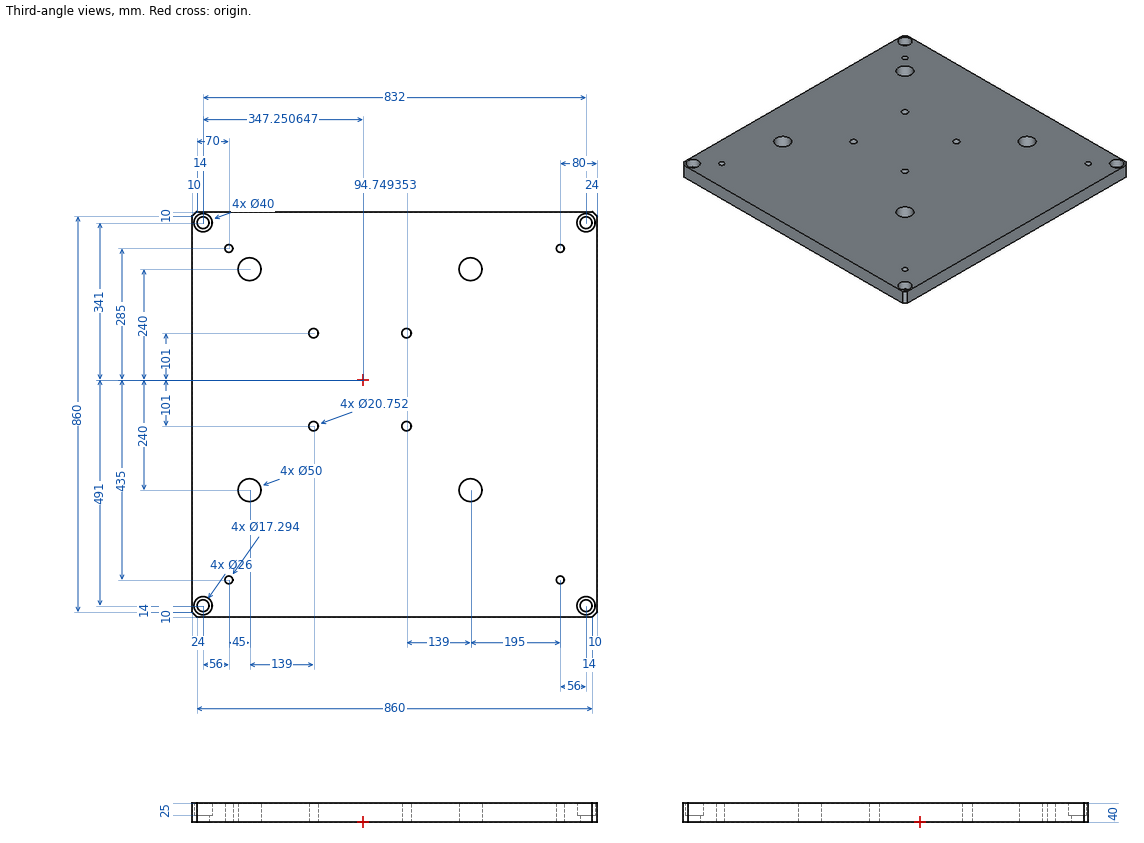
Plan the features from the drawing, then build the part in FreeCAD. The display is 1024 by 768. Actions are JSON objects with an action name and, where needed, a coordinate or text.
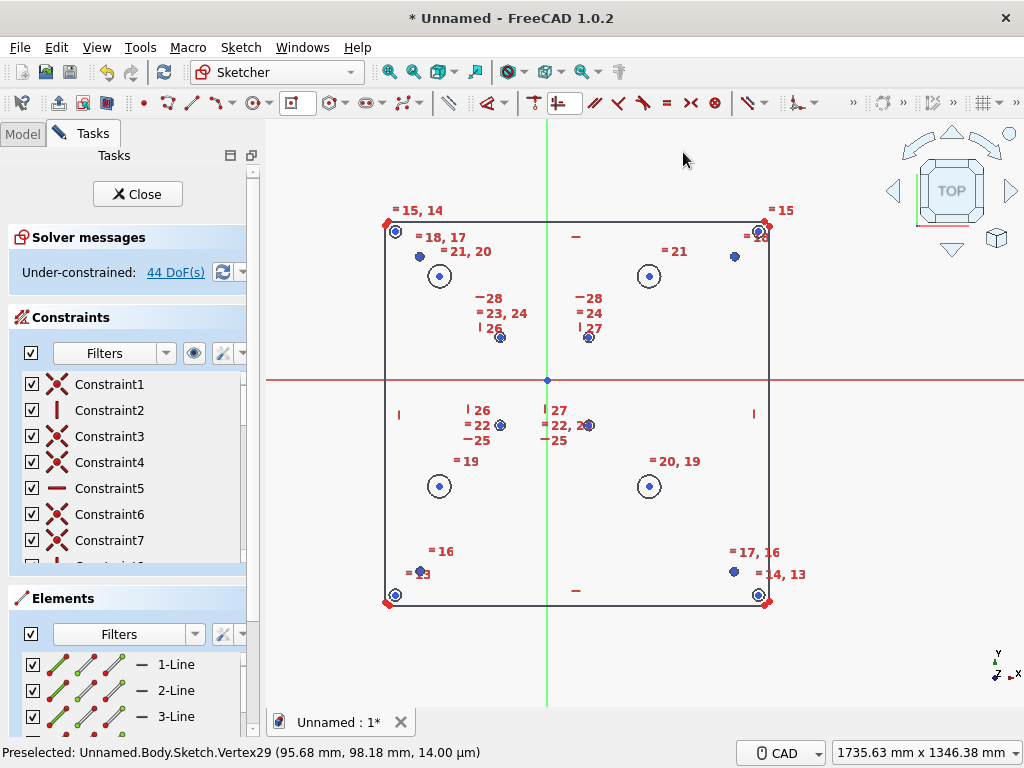
{"action": "scroll", "coordinate": [400, 599], "scroll_direction": "up", "scroll_amount": 7}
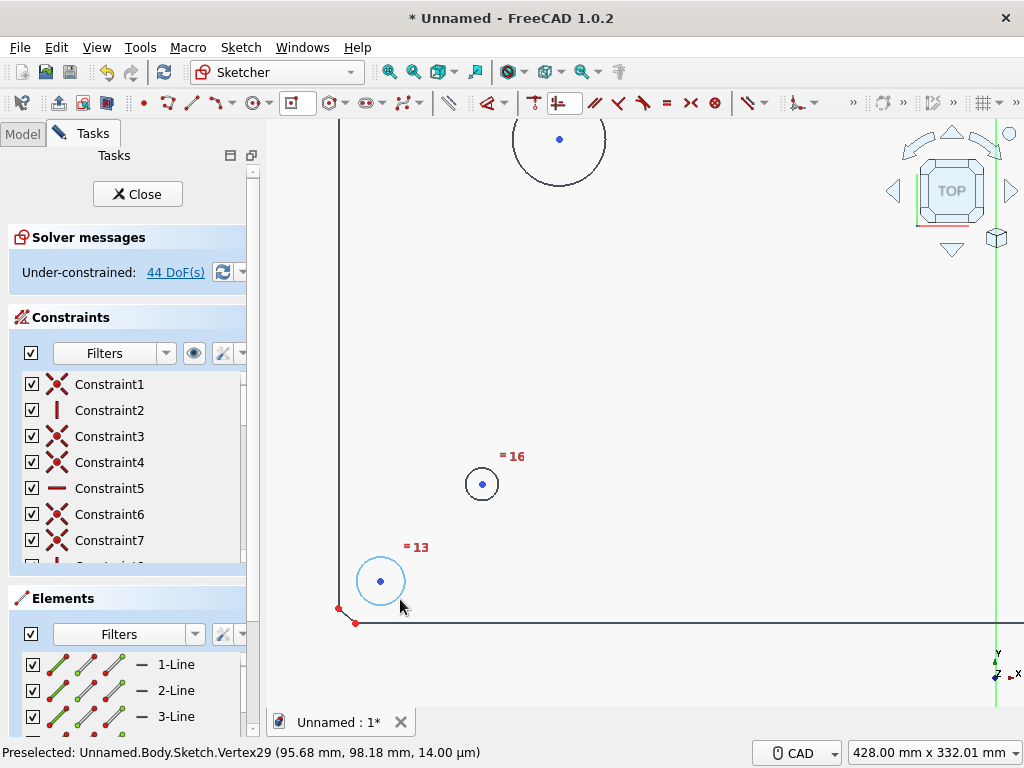
{"action": "left_click", "coordinate": [398, 598]}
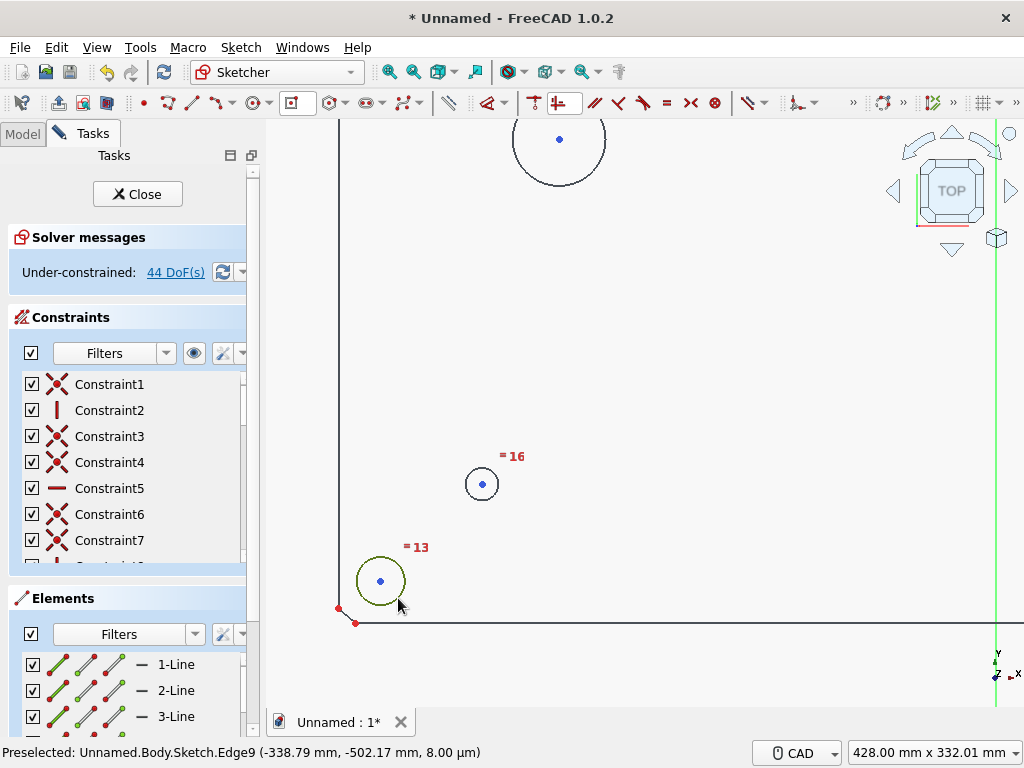
{"action": "left_click", "coordinate": [506, 104]}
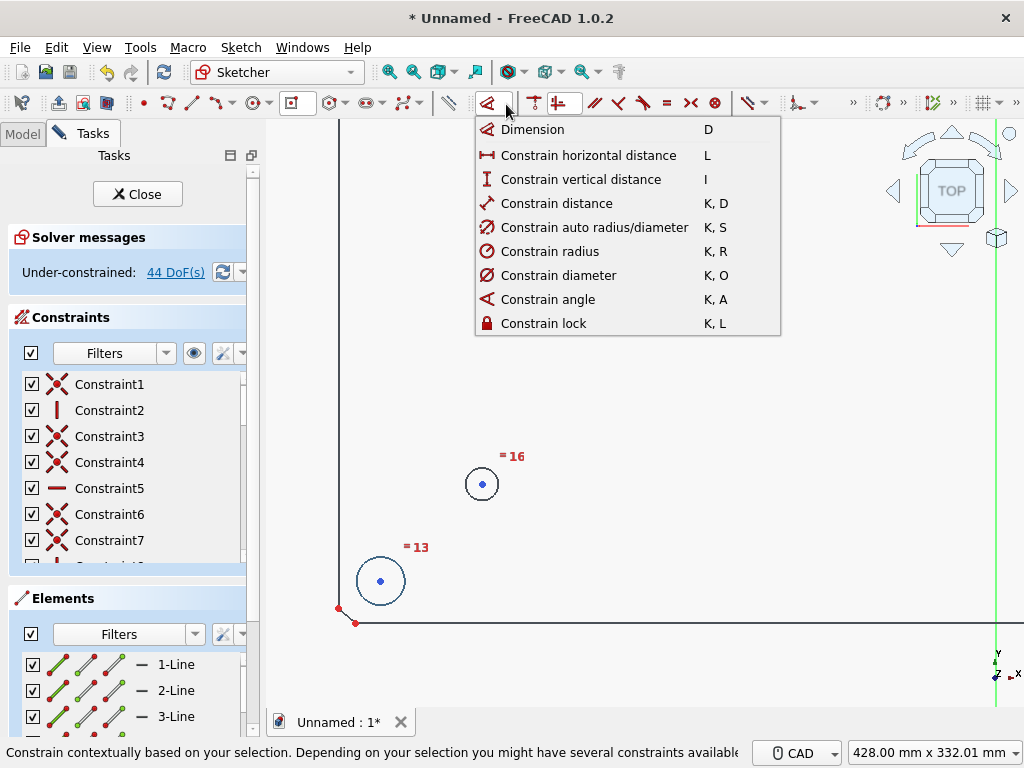
{"action": "left_click", "coordinate": [628, 275]}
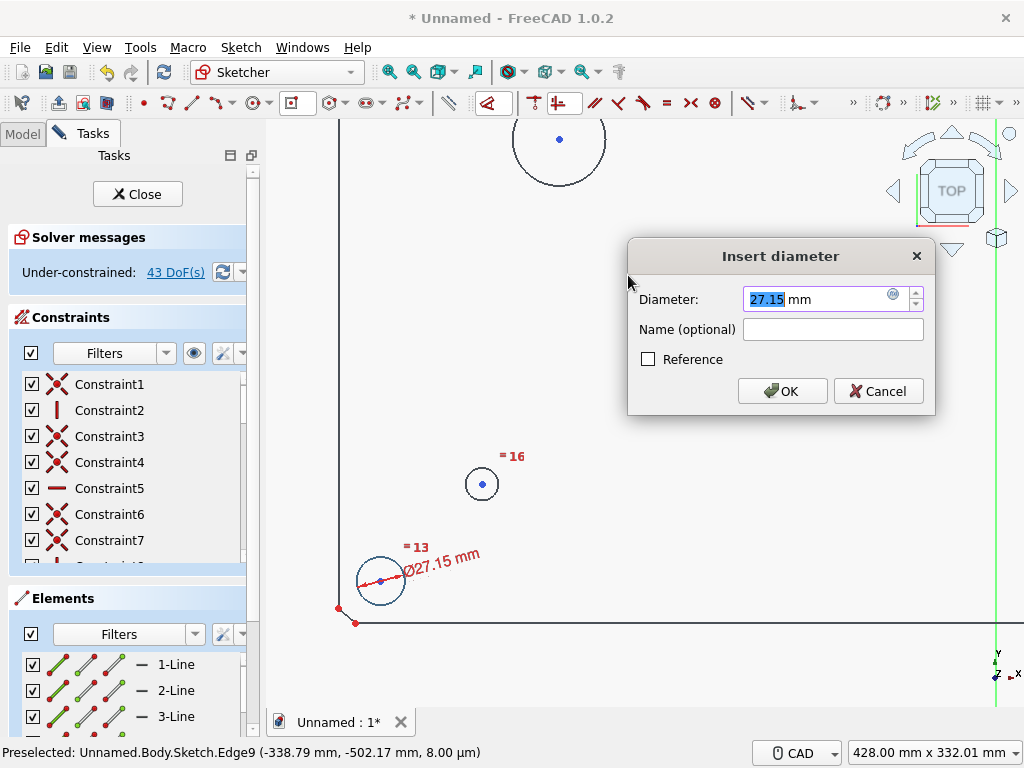
{"action": "type", "text": "26"}
{"action": "key", "text": "Return"}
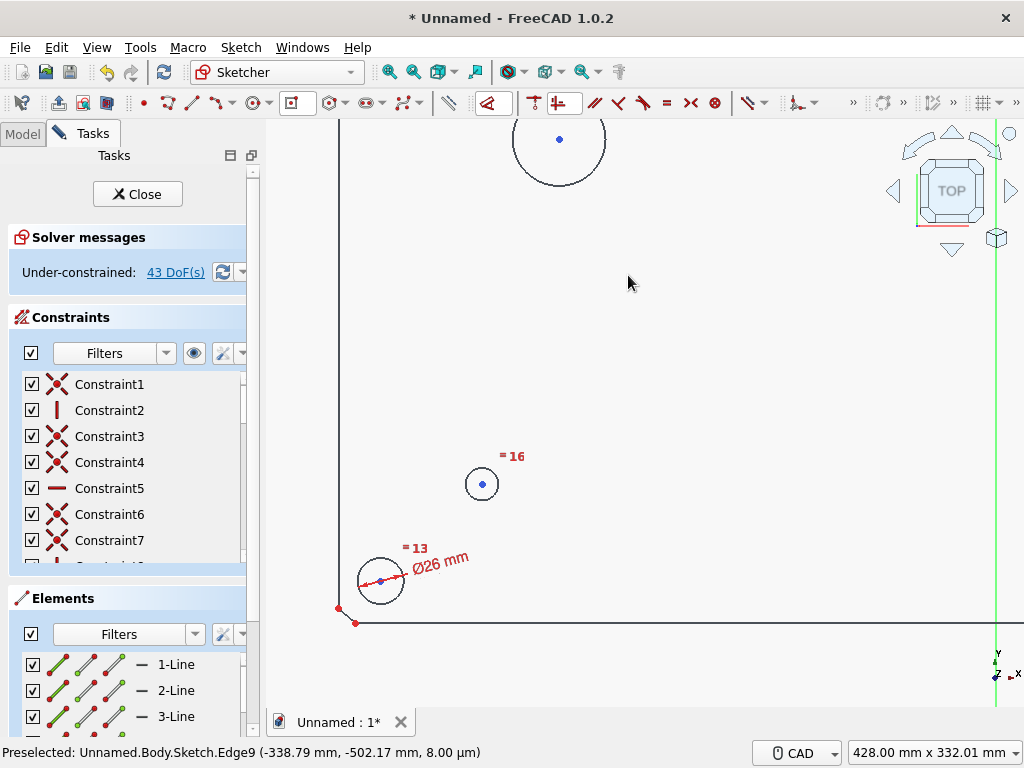
{"action": "scroll", "coordinate": [494, 473], "scroll_direction": "up", "scroll_amount": 2}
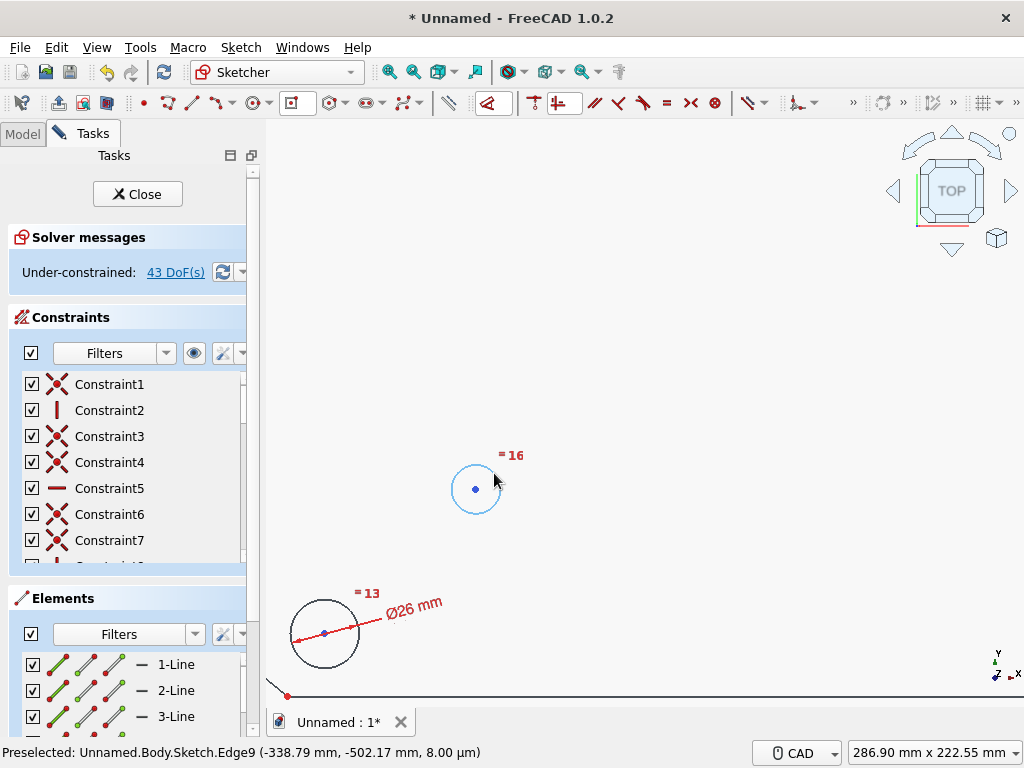
{"action": "left_click", "coordinate": [493, 472]}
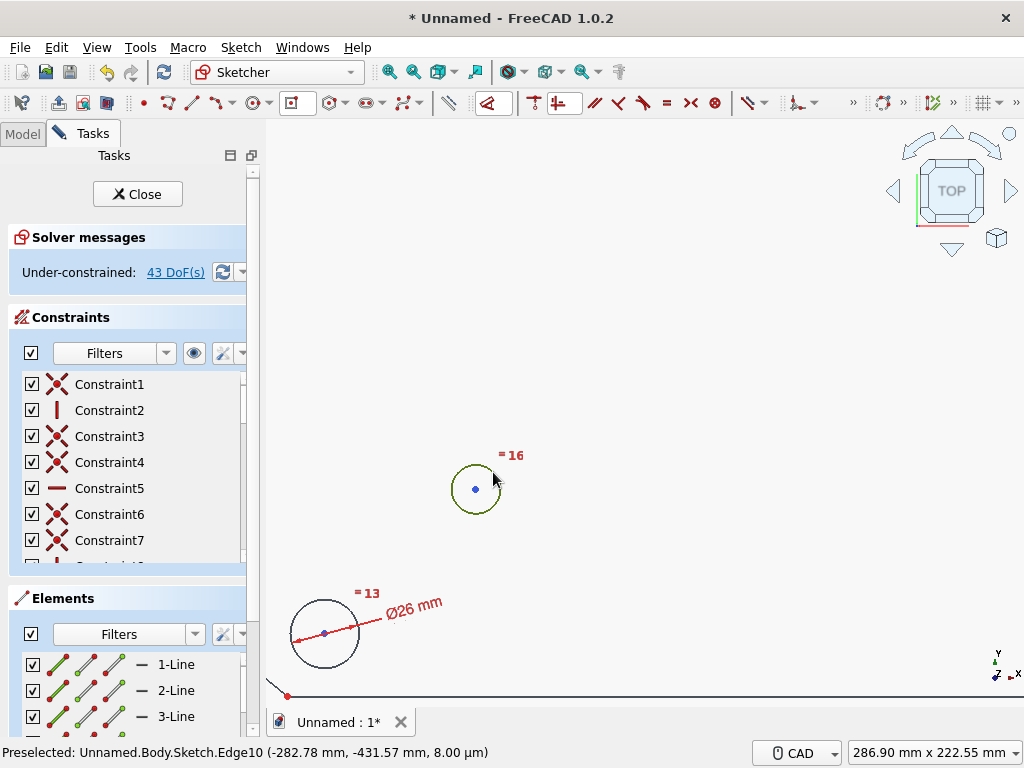
{"action": "key", "text": "k o"}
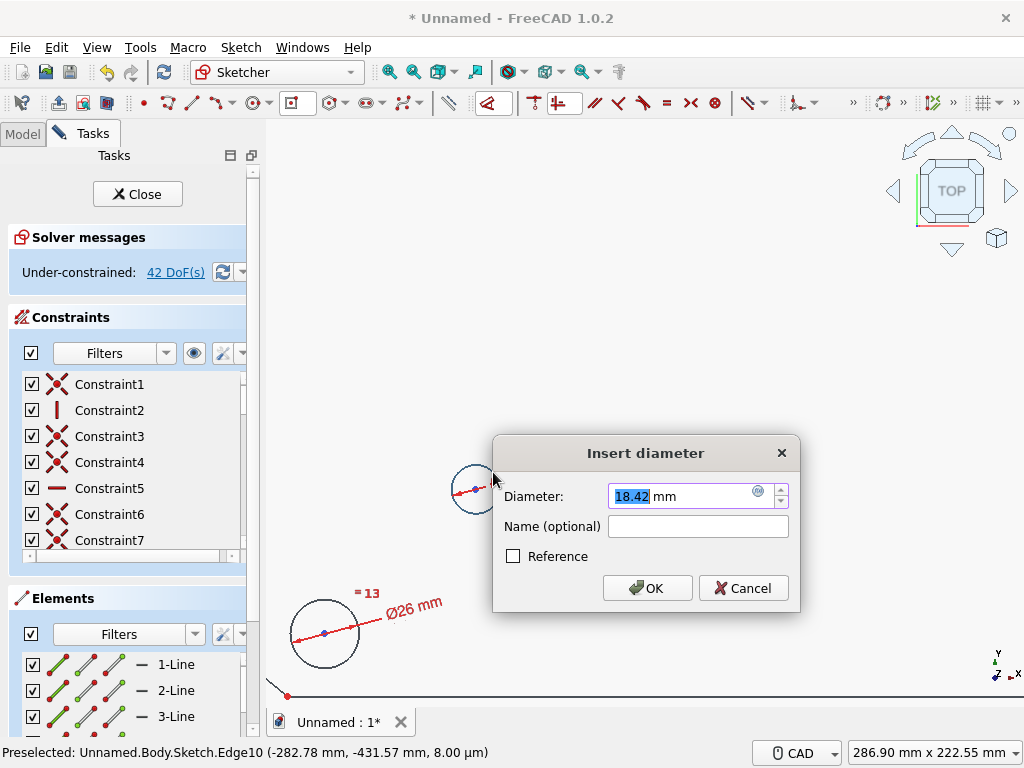
{"action": "type", "text": "17.294"}
{"action": "key", "text": "Return"}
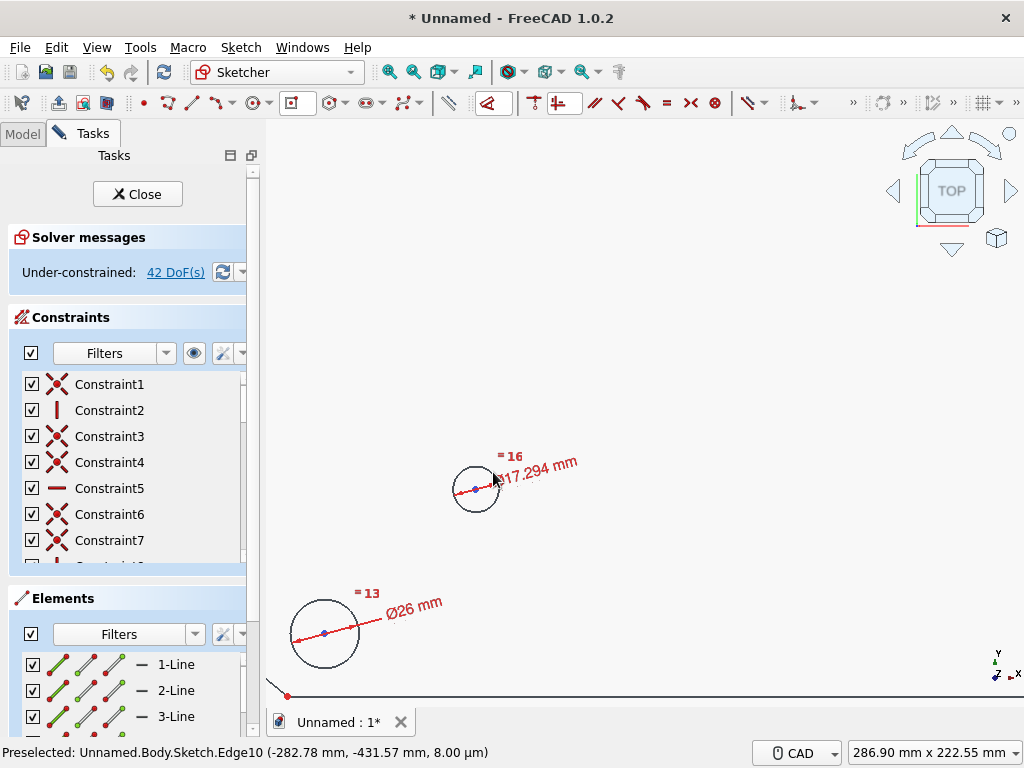
{"action": "scroll", "coordinate": [409, 587], "scroll_direction": "down", "scroll_amount": 9}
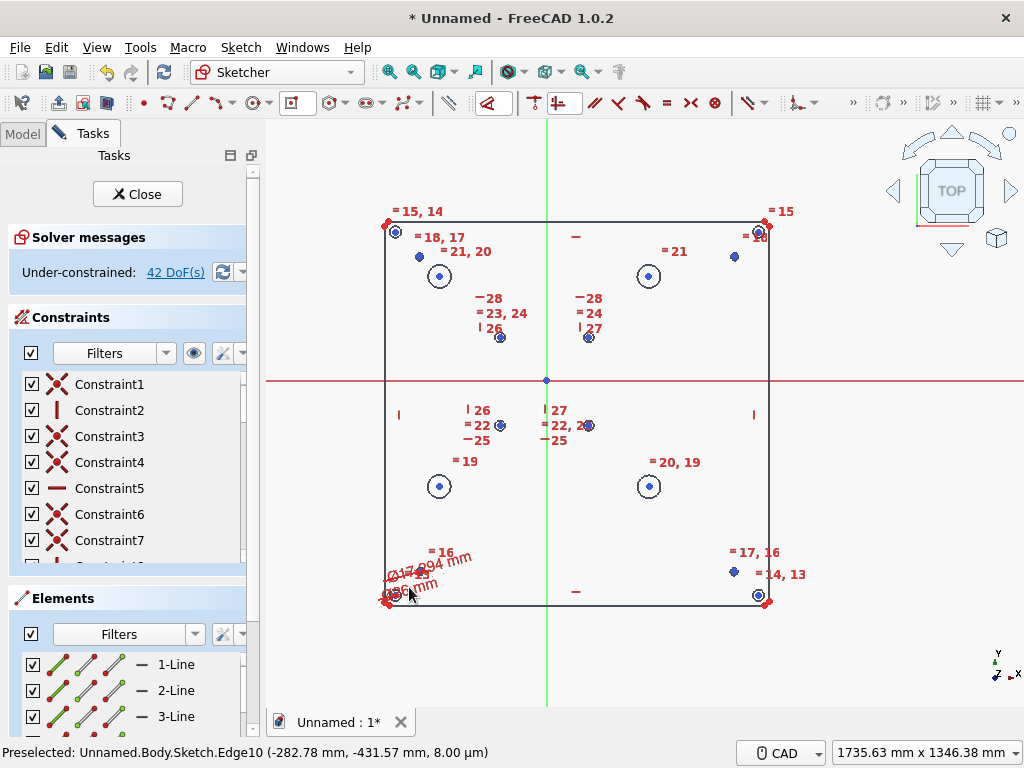
{"action": "scroll", "coordinate": [447, 478], "scroll_direction": "up", "scroll_amount": 3}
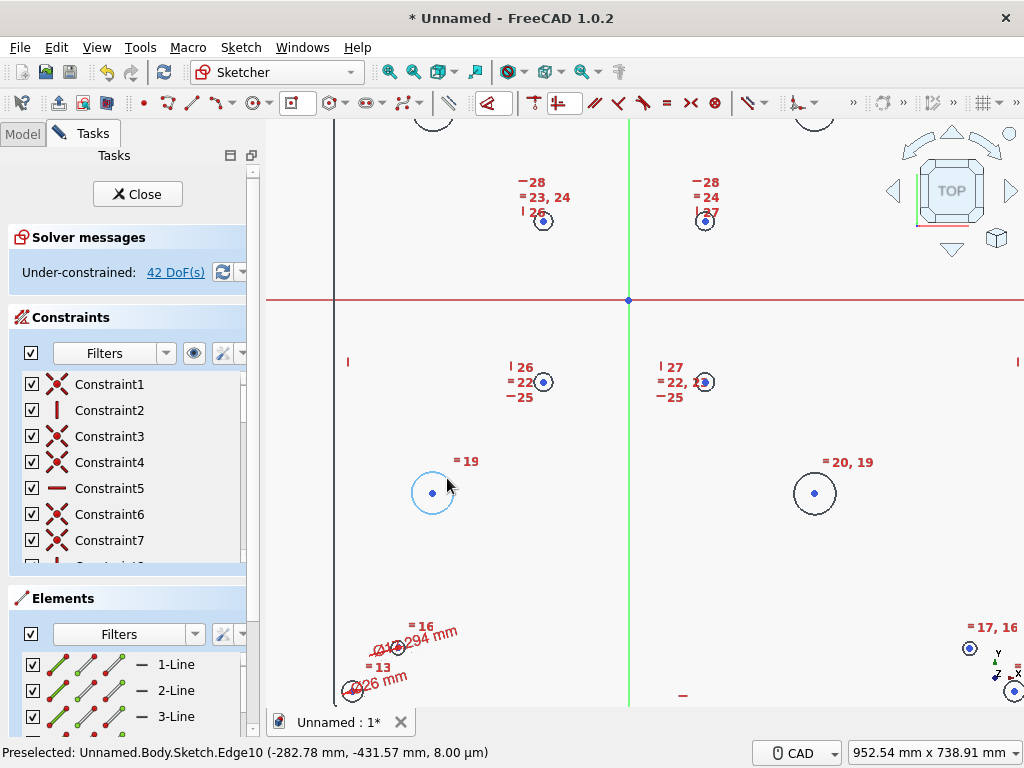
{"action": "left_click", "coordinate": [447, 478]}